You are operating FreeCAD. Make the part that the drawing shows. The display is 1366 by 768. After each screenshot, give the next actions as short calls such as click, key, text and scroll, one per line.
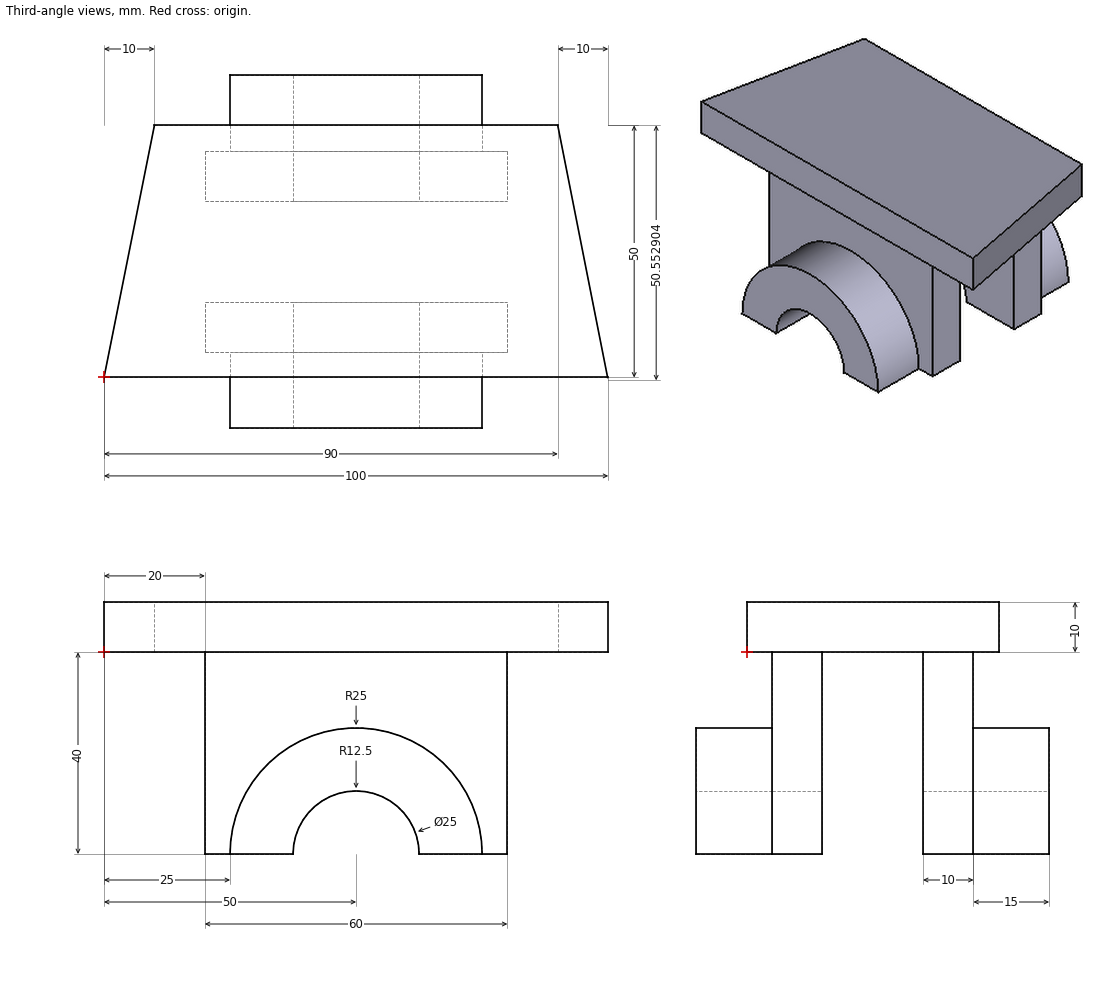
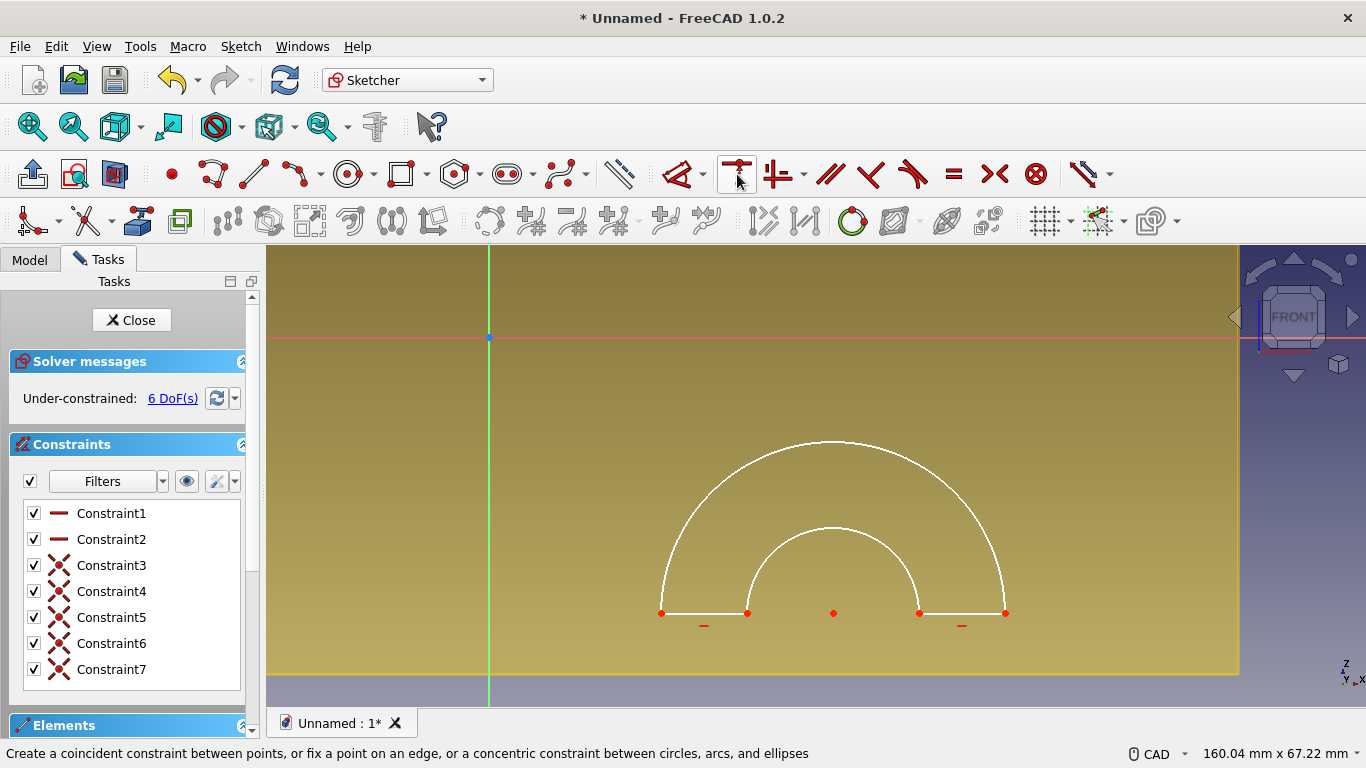
click(934, 475)
click(953, 449)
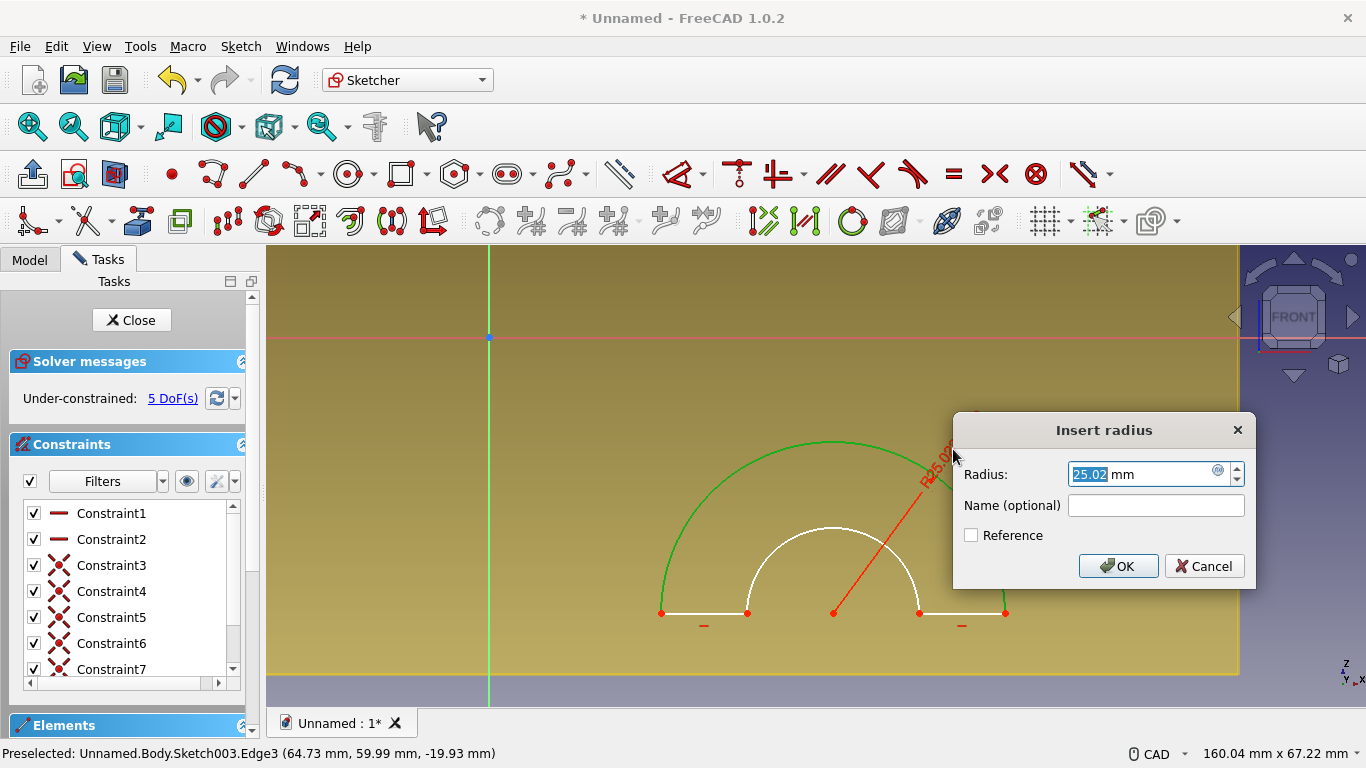
text(25)
key(Return)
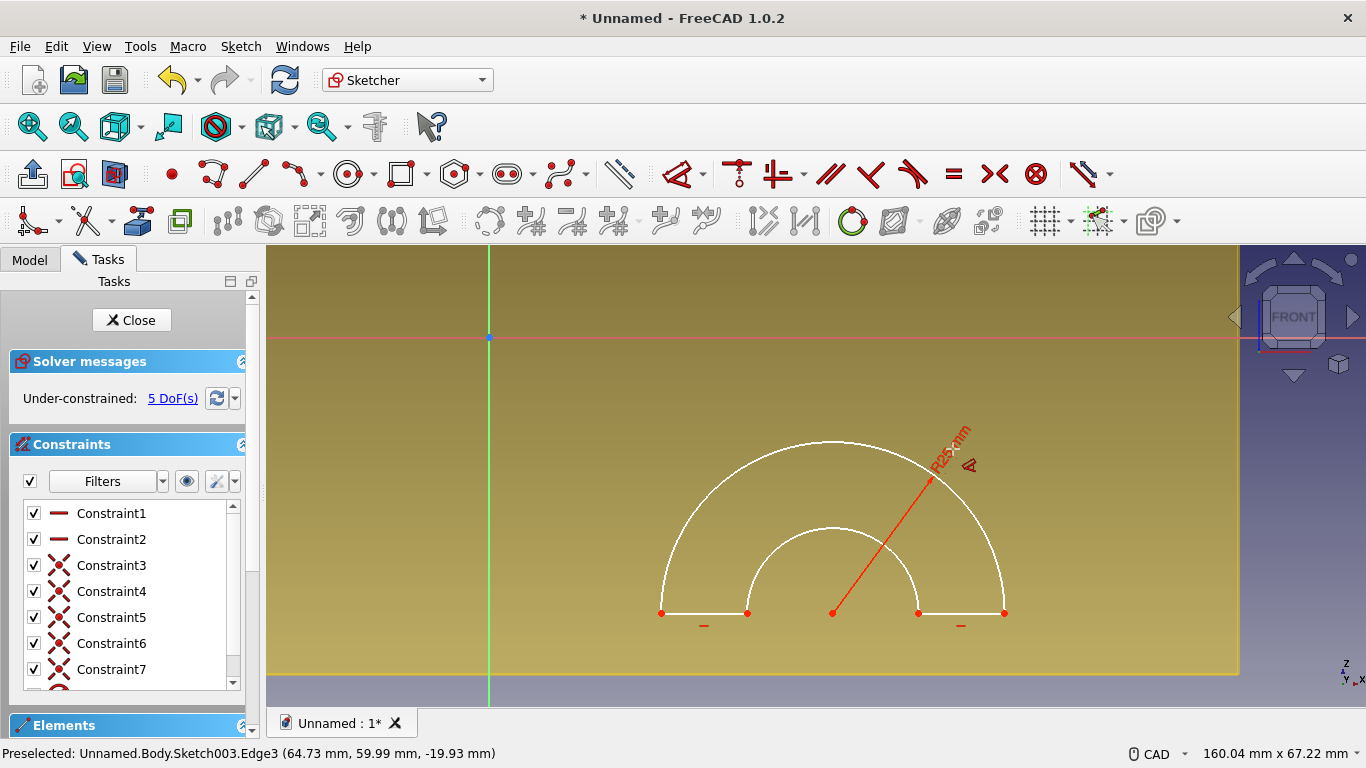
click(883, 545)
click(902, 519)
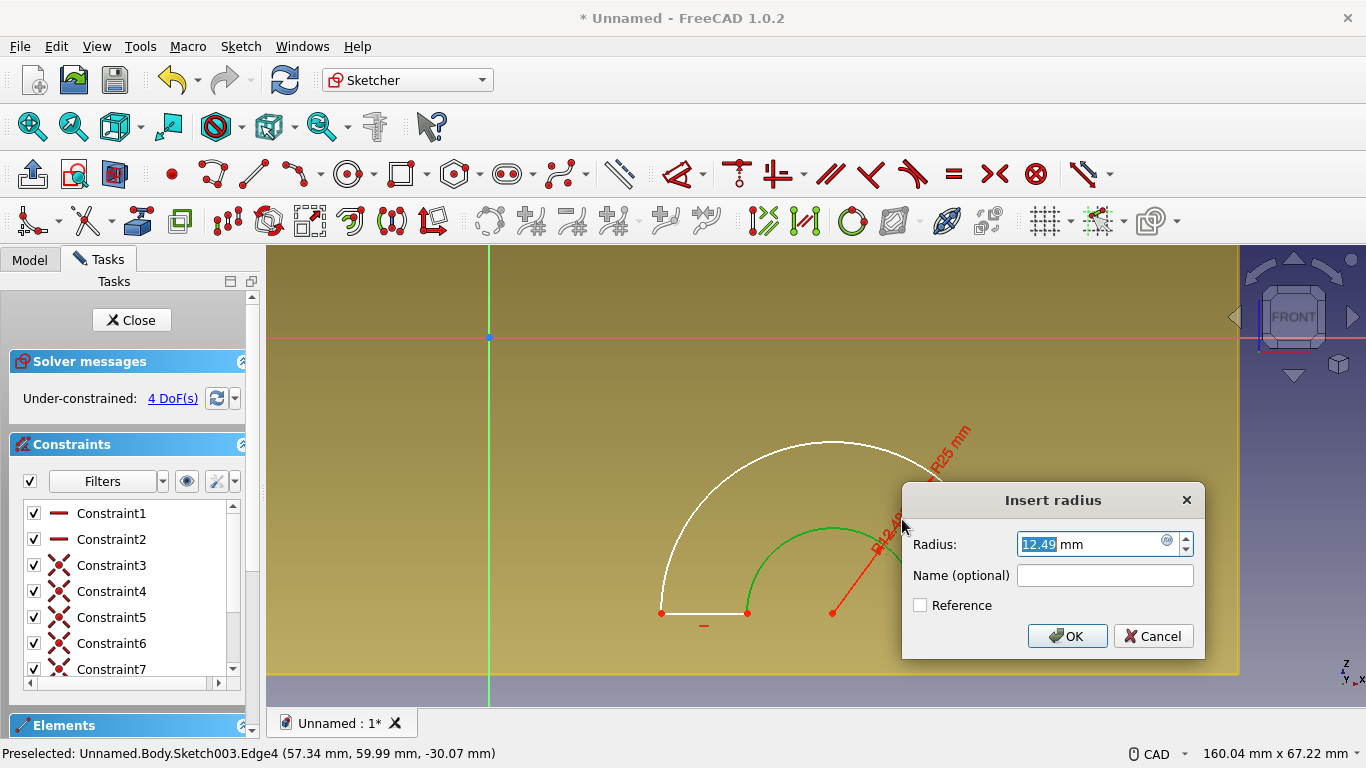
text(12.5)
key(Return)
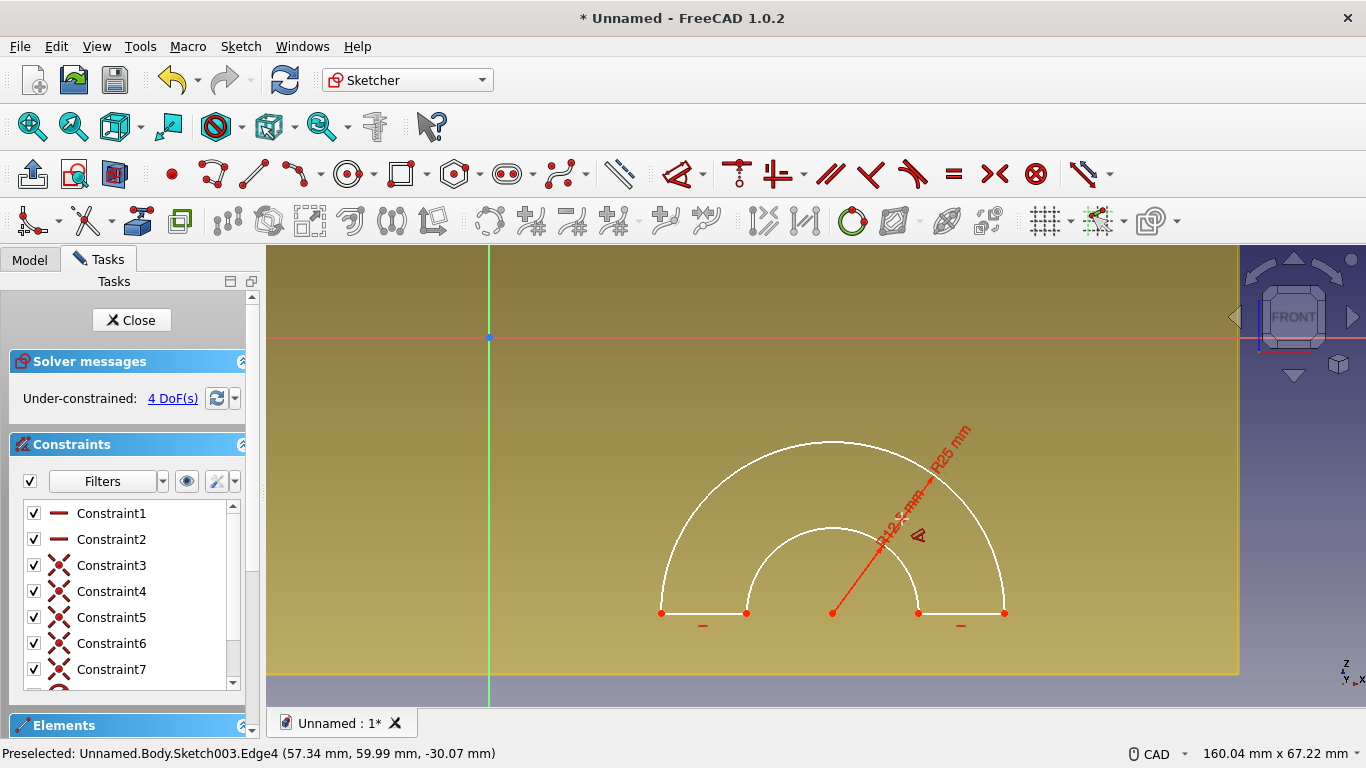
click(747, 614)
click(455, 476)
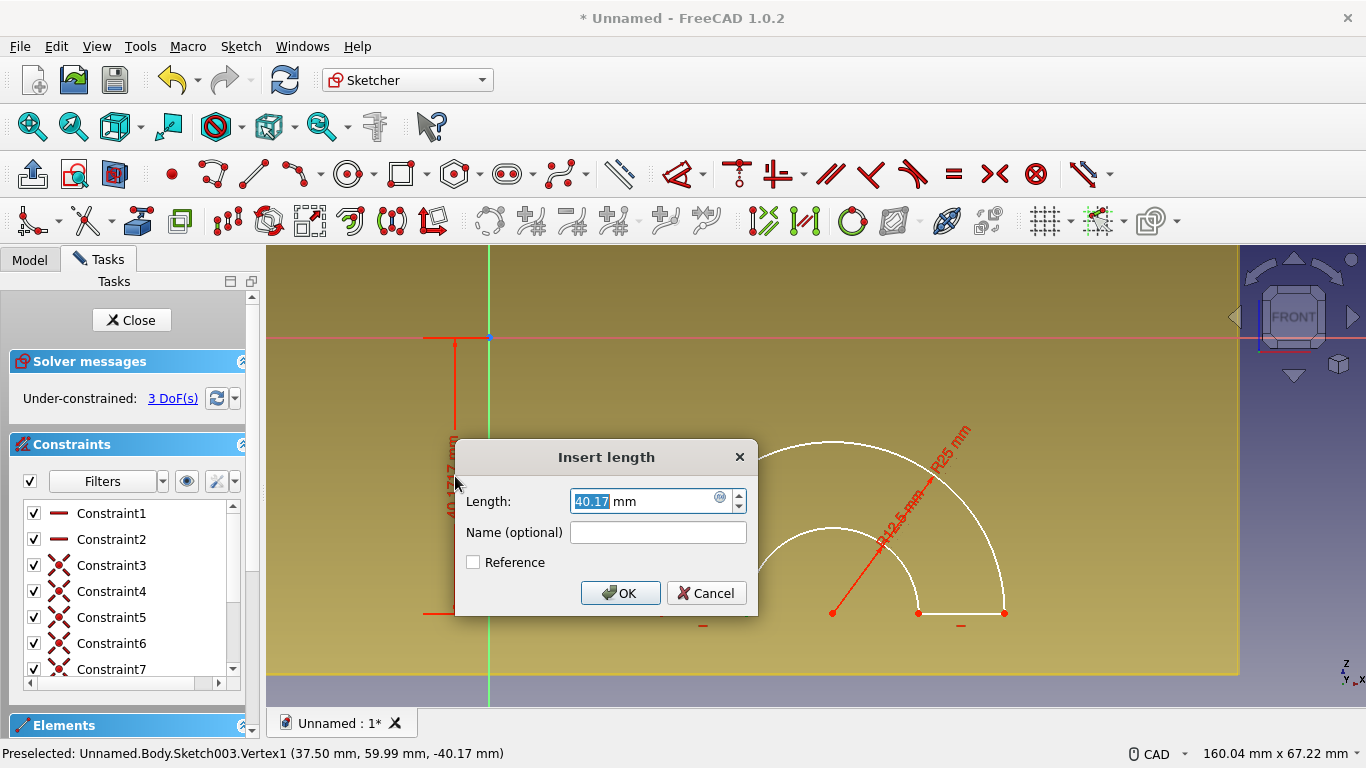
text(40)
key(Return)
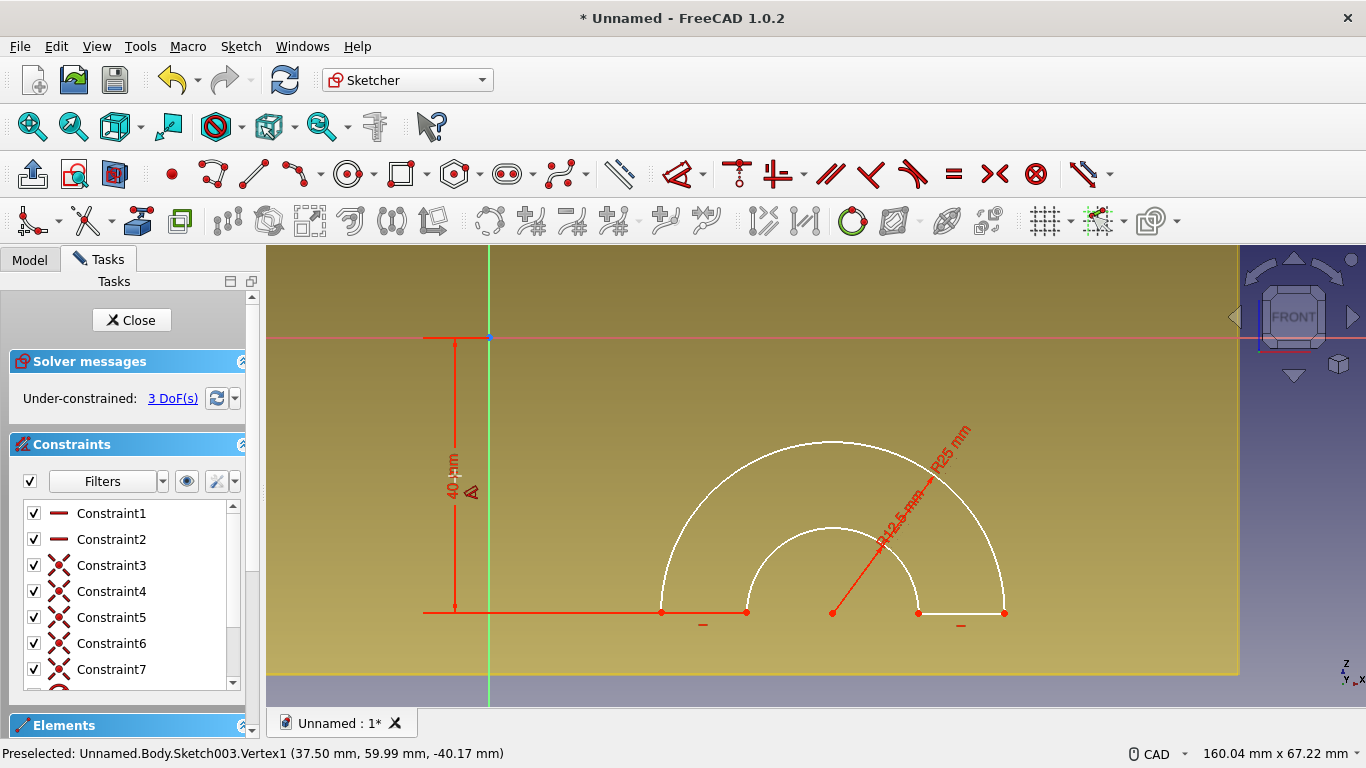
click(661, 613)
click(575, 647)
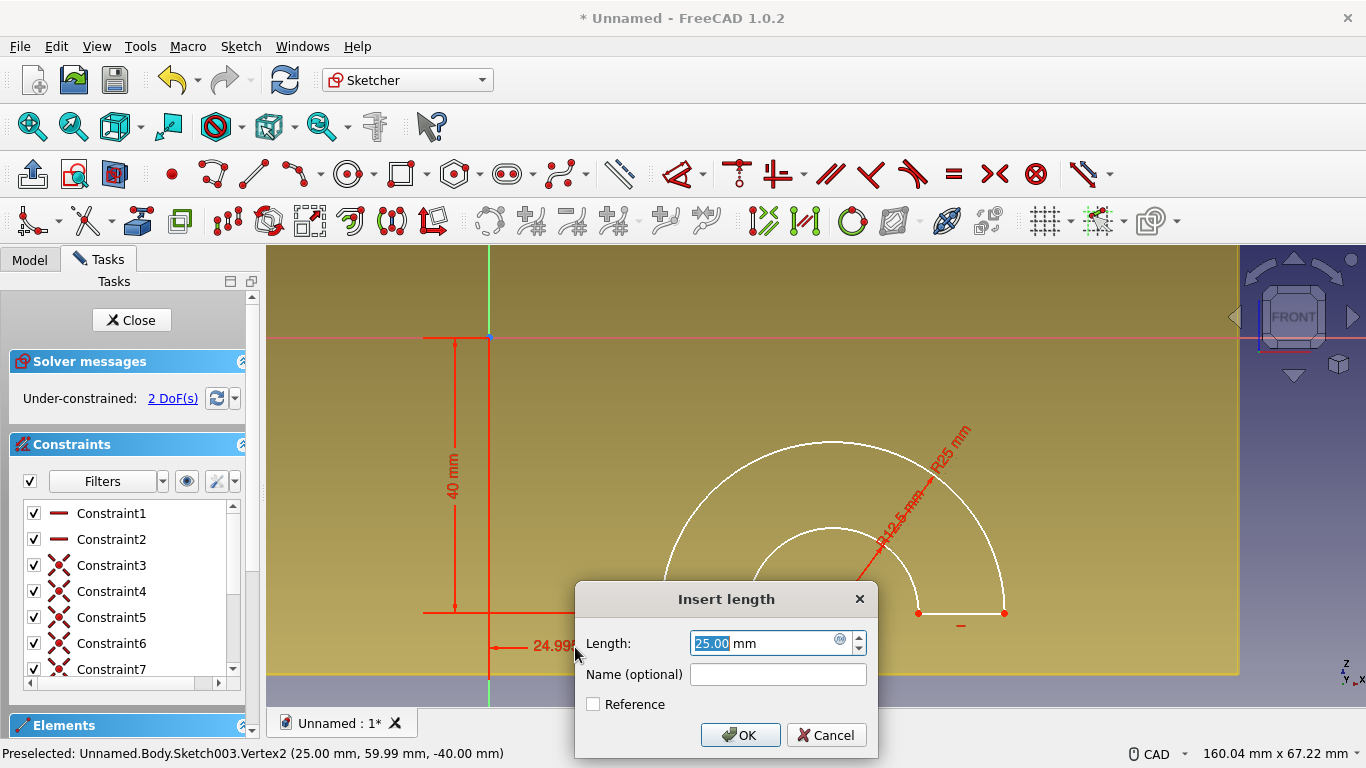
text(25)
key(Return)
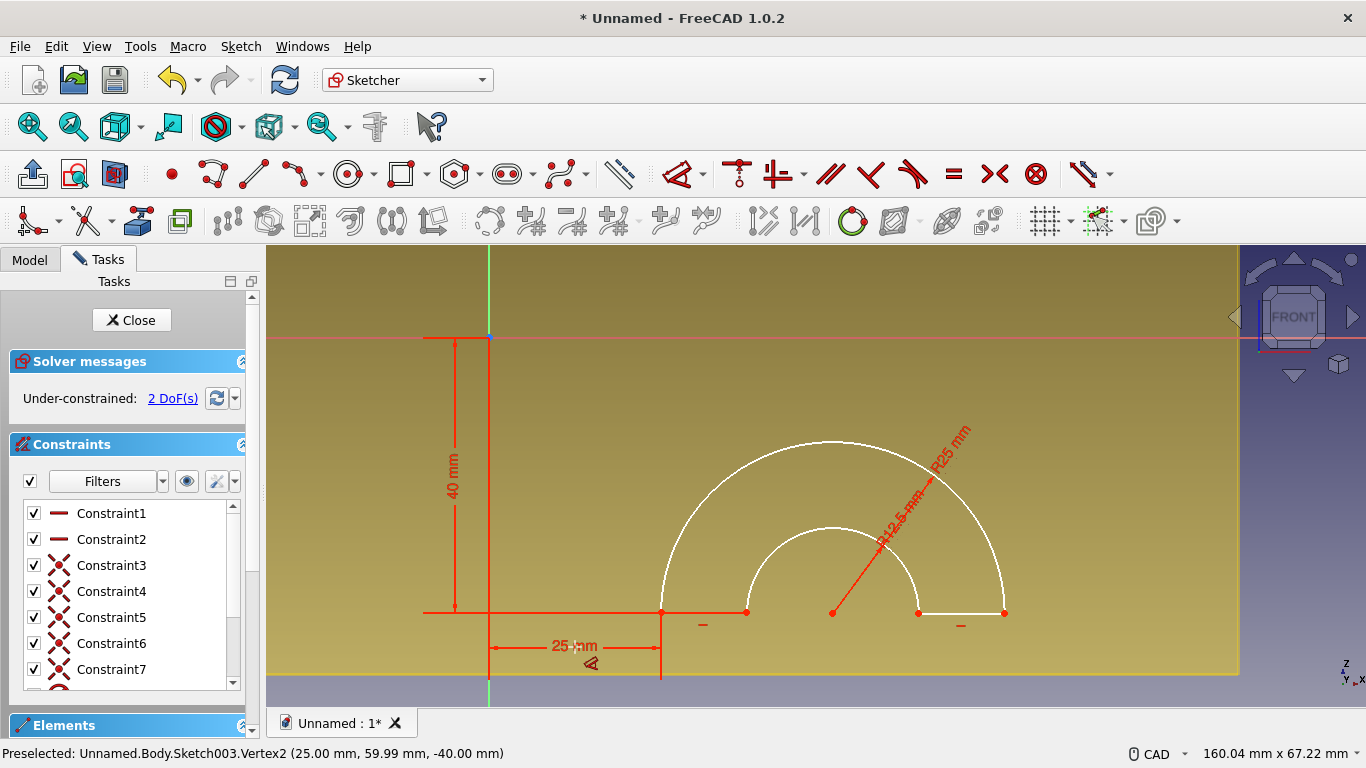
click(1005, 614)
click(455, 412)